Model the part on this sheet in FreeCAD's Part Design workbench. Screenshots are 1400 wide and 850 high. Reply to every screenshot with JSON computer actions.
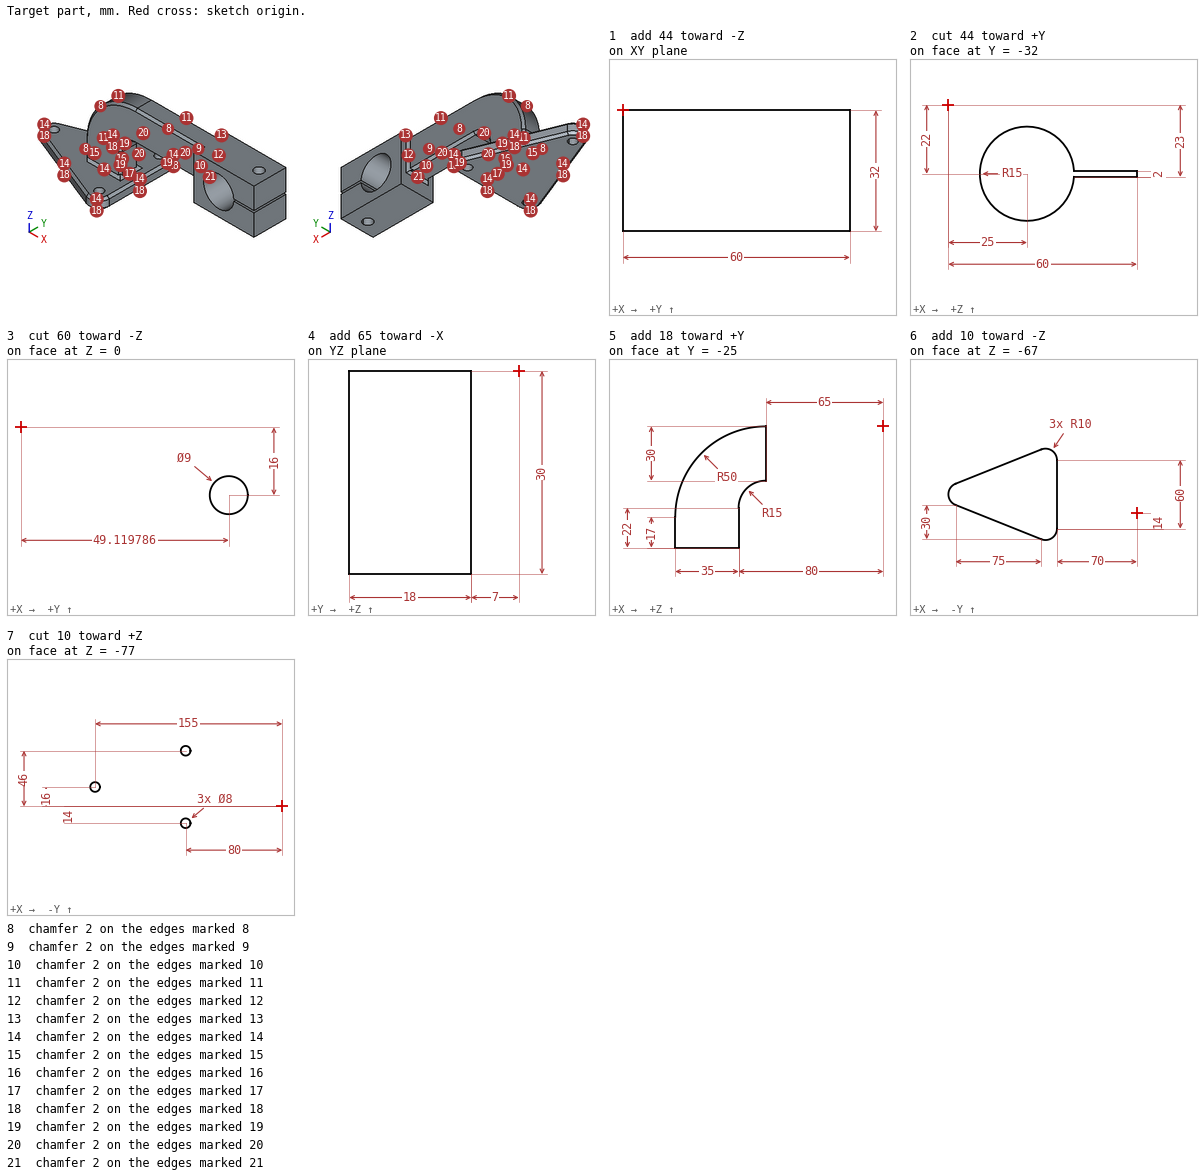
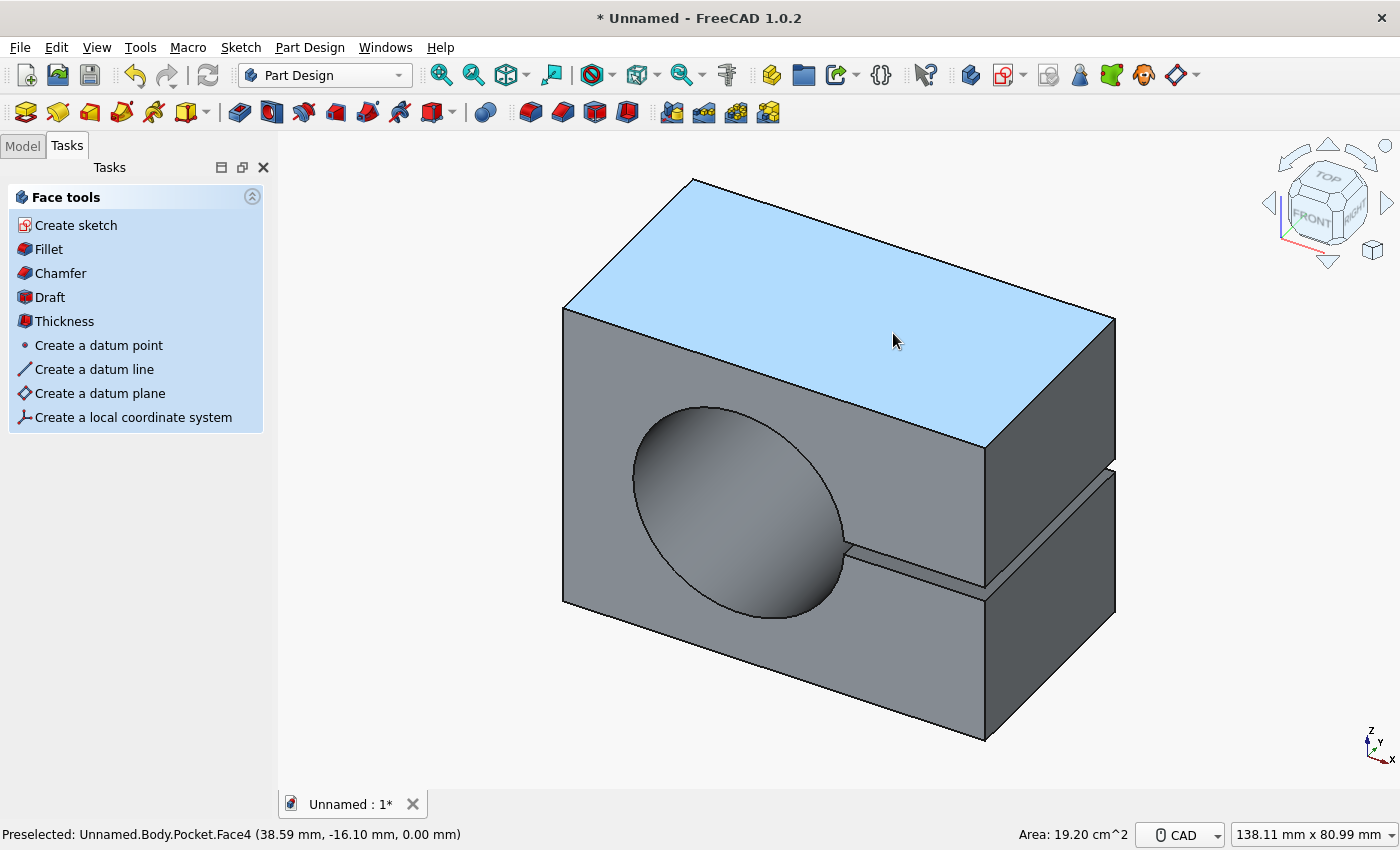
{"action": "left_click", "coordinate": [1004, 76]}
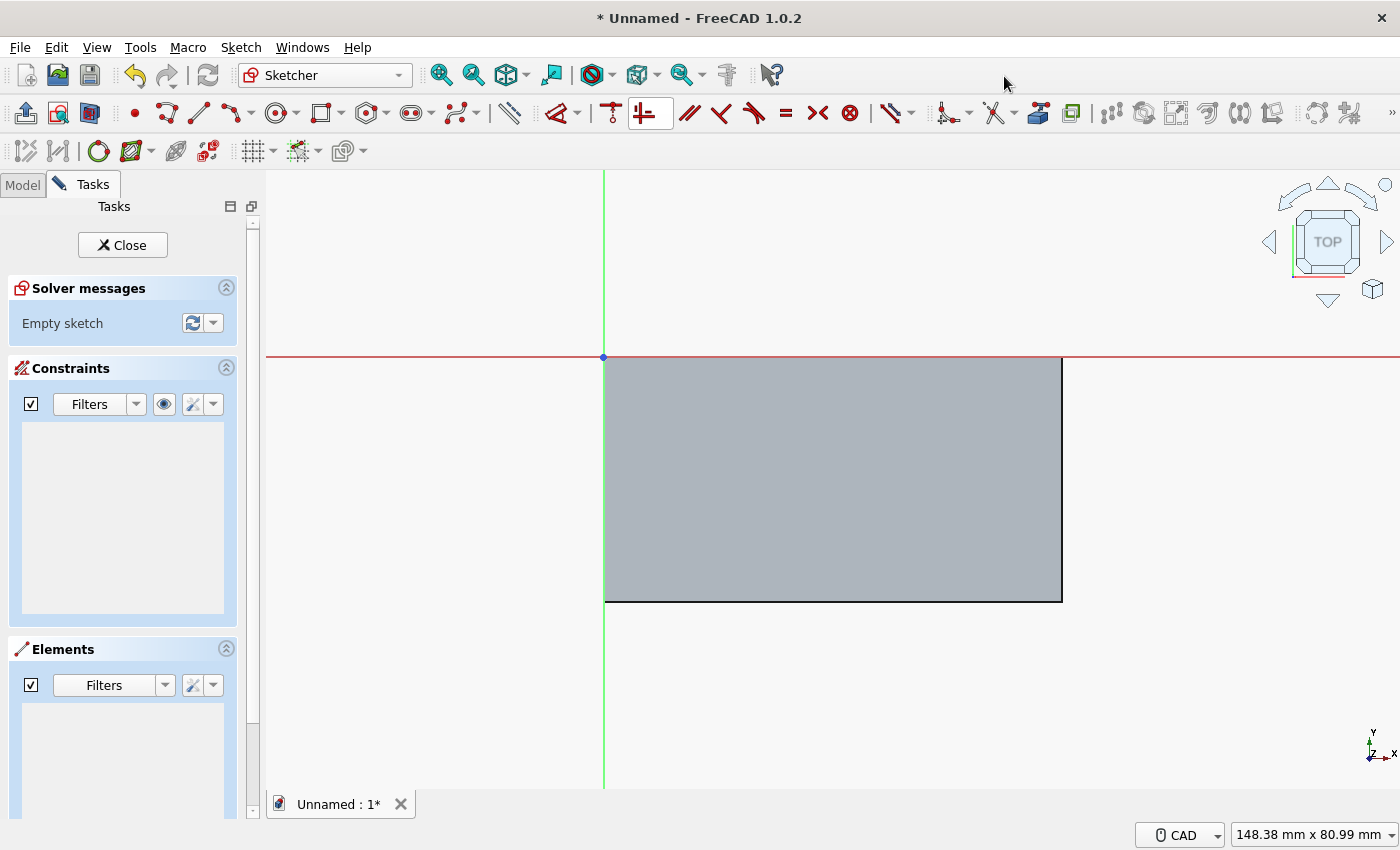
{"action": "scroll", "coordinate": [1022, 479], "scroll_direction": "up", "scroll_amount": 9}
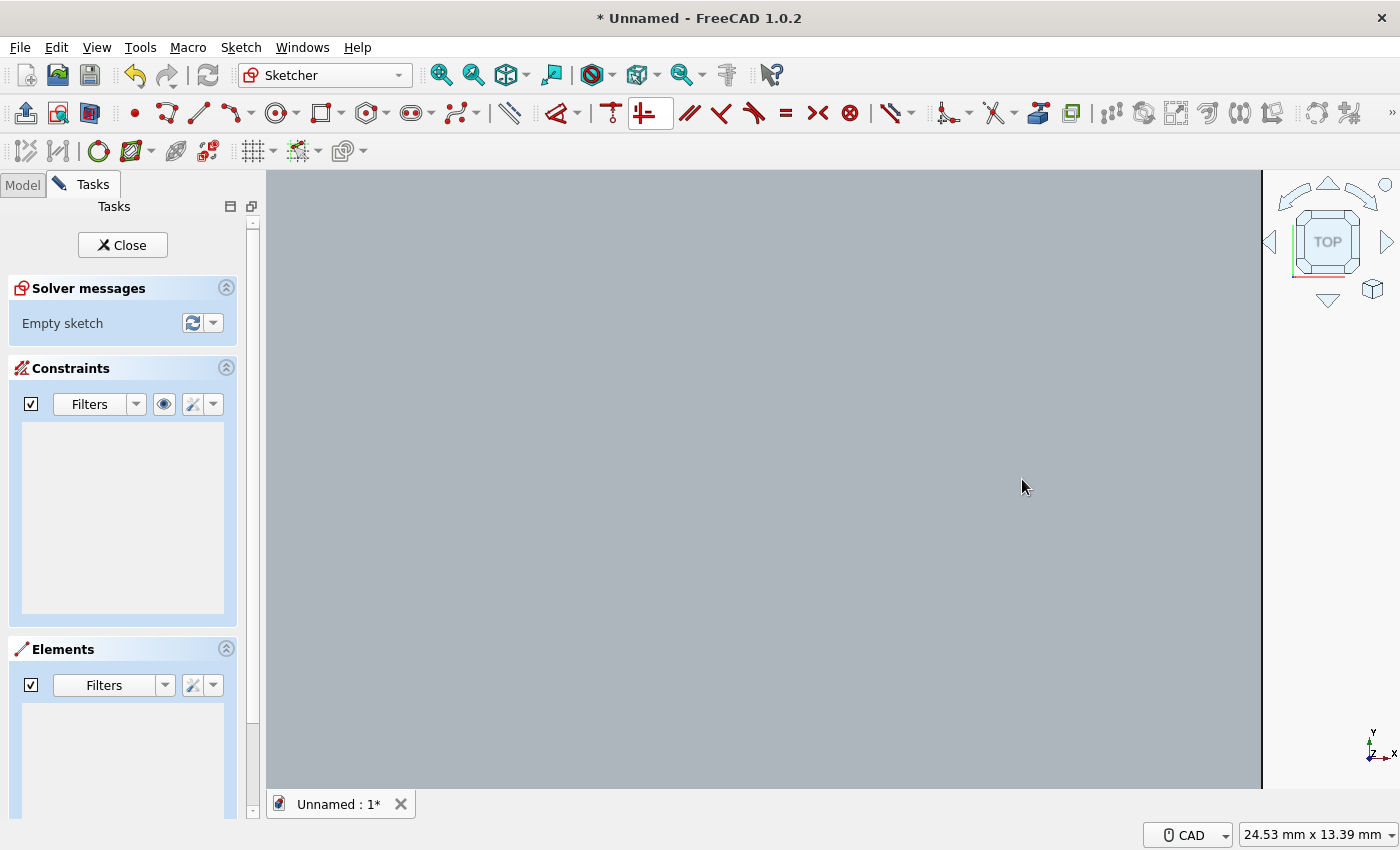
{"action": "left_click", "coordinate": [276, 114]}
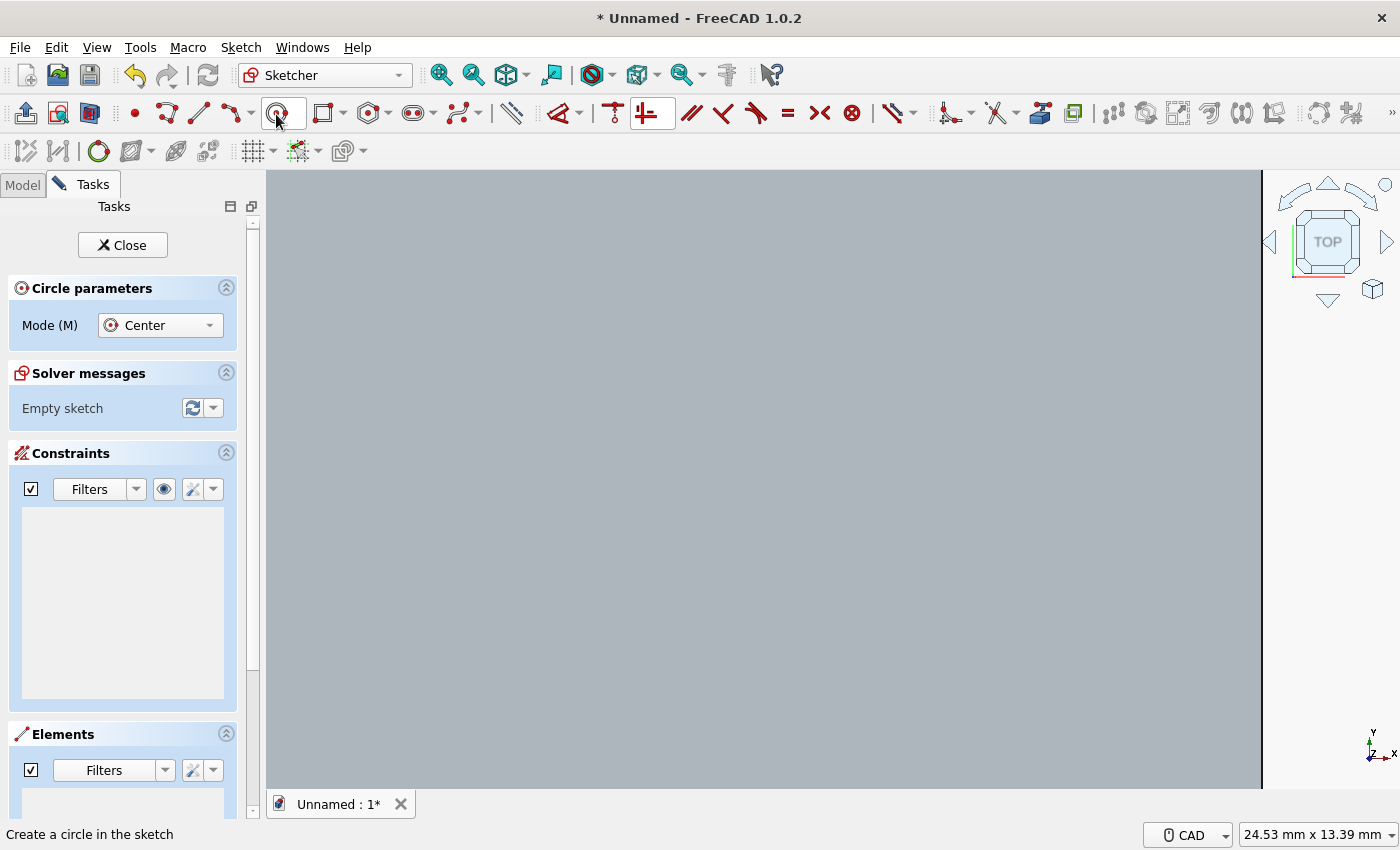
{"action": "left_click", "coordinate": [759, 479]}
{"action": "mouse_move", "coordinate": [906, 332]}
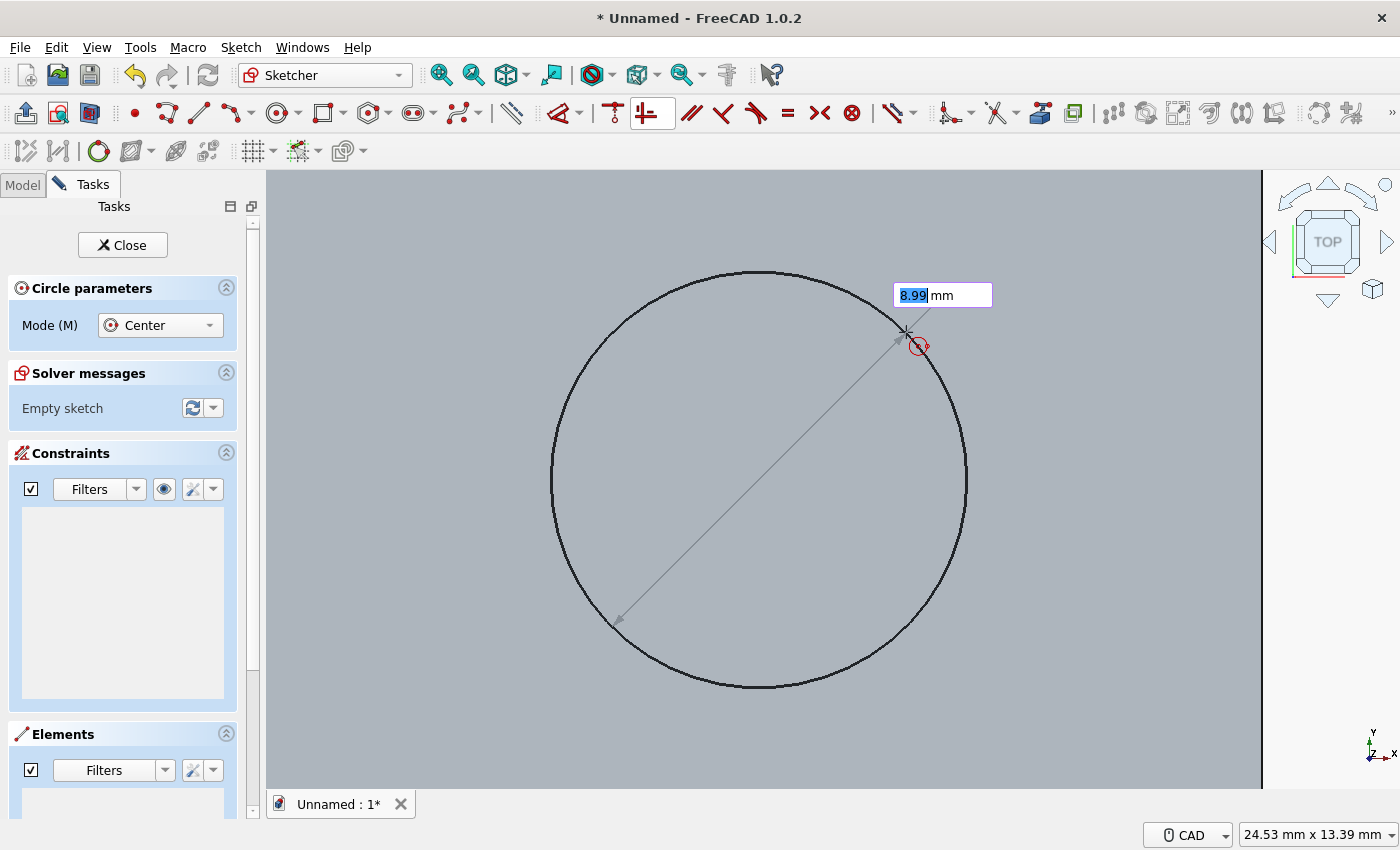
{"action": "type", "text": "9"}
{"action": "key", "text": "Return"}
{"action": "key", "text": "Escape"}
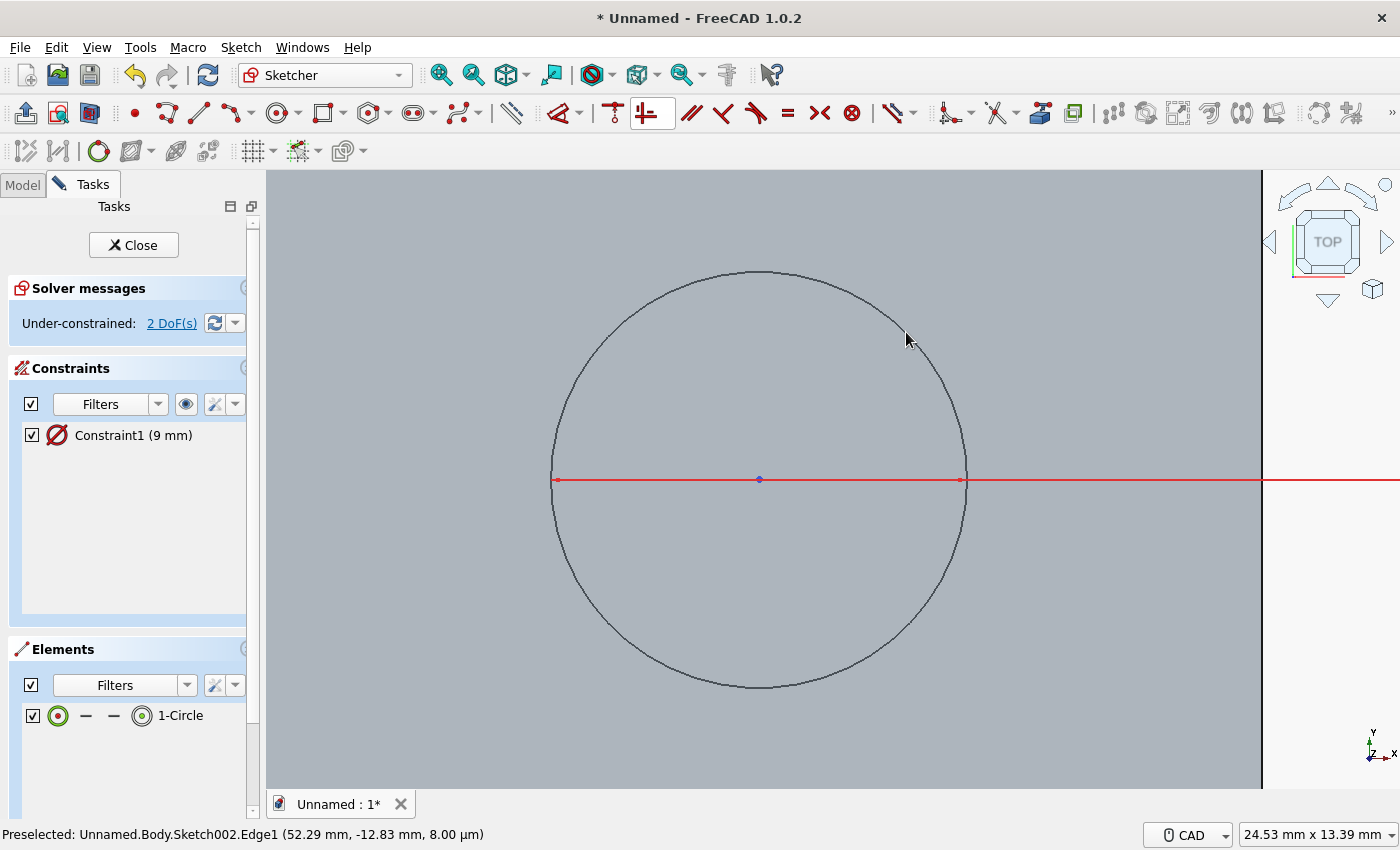
{"action": "left_click", "coordinate": [558, 114]}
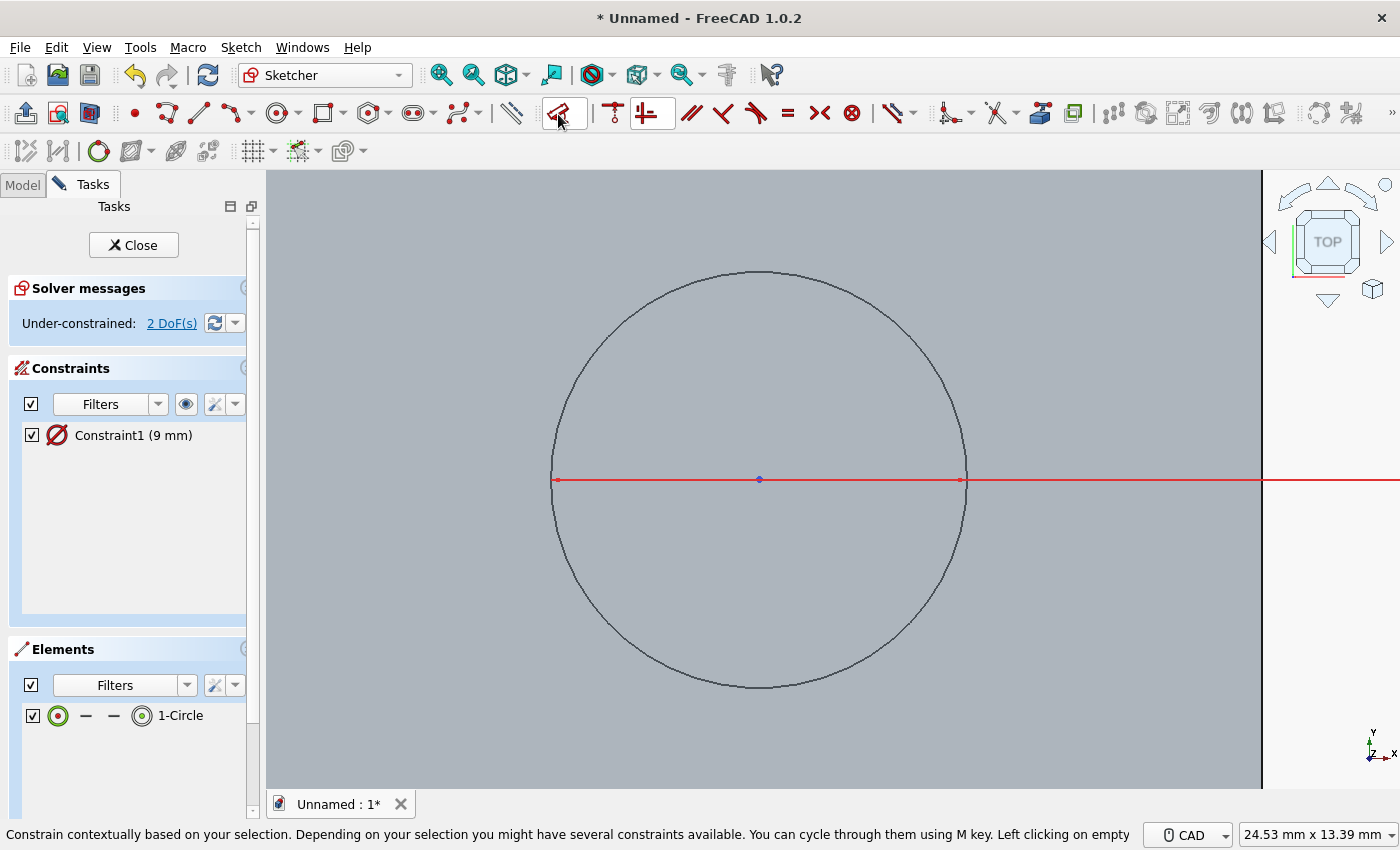
{"action": "left_click", "coordinate": [759, 480]}
{"action": "left_click", "coordinate": [793, 339]}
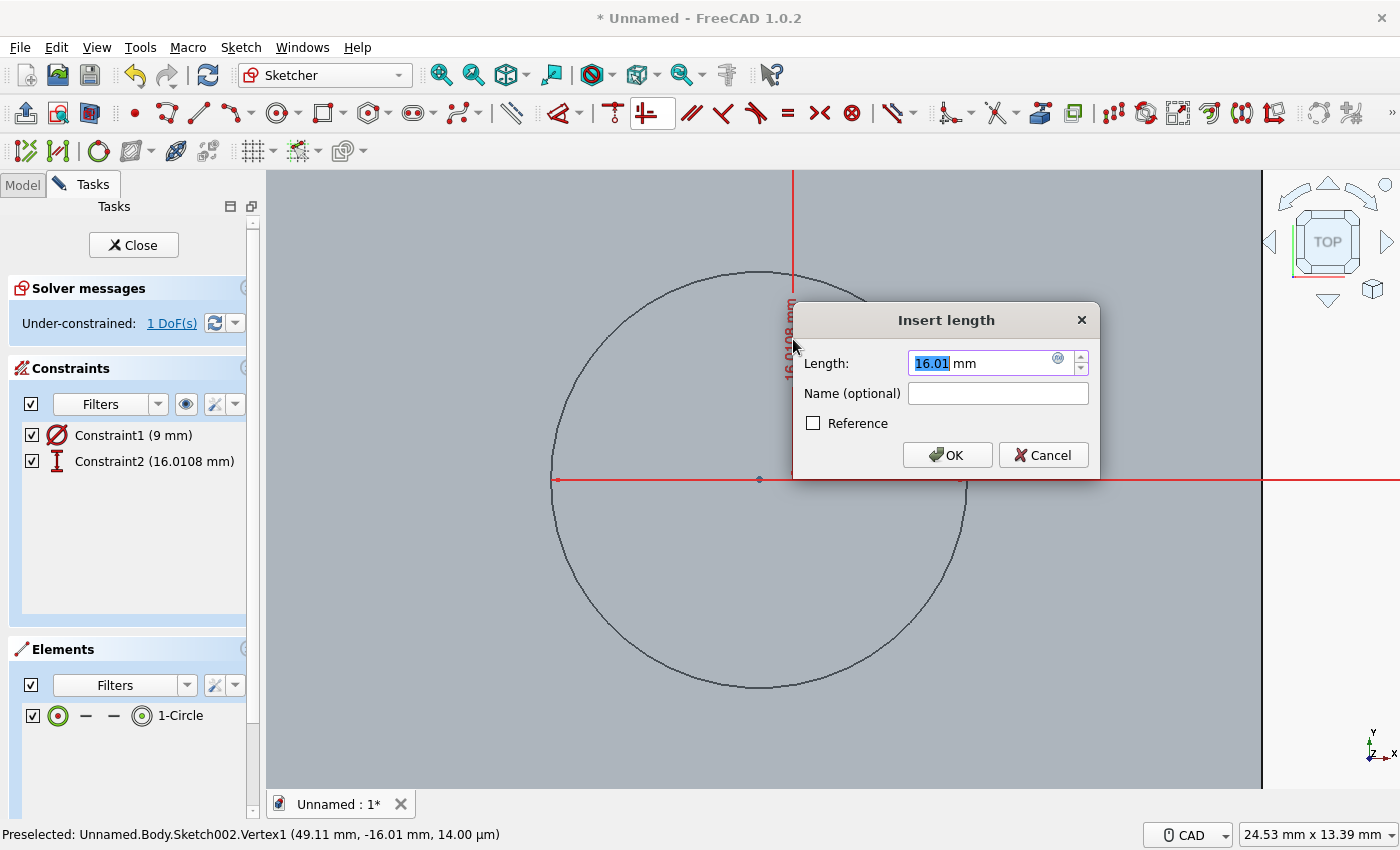
{"action": "type", "text": "16"}
{"action": "key", "text": "Return"}